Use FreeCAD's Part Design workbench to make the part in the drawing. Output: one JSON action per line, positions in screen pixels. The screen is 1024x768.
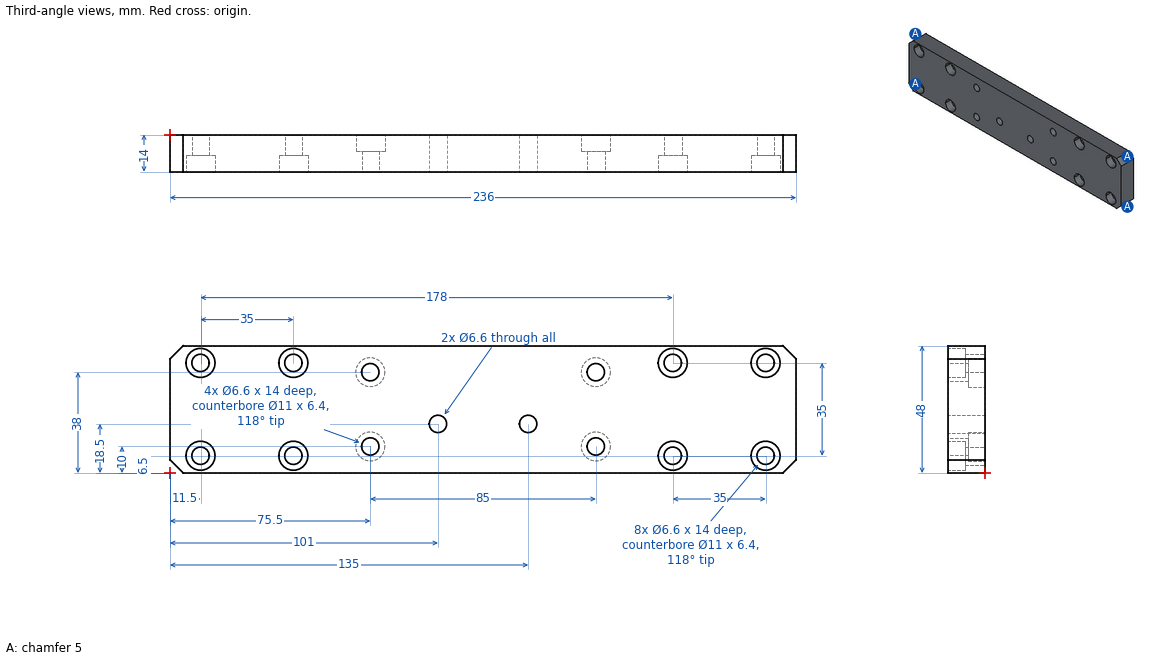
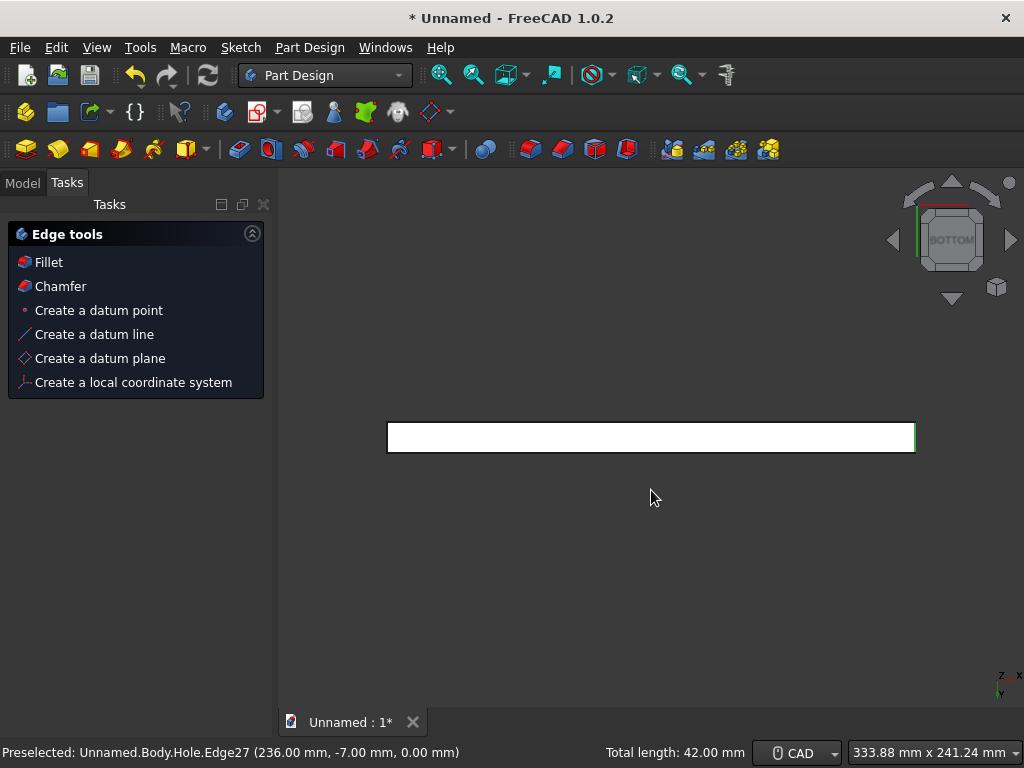
{"action": "left_click", "coordinate": [387, 436], "text": "ctrl"}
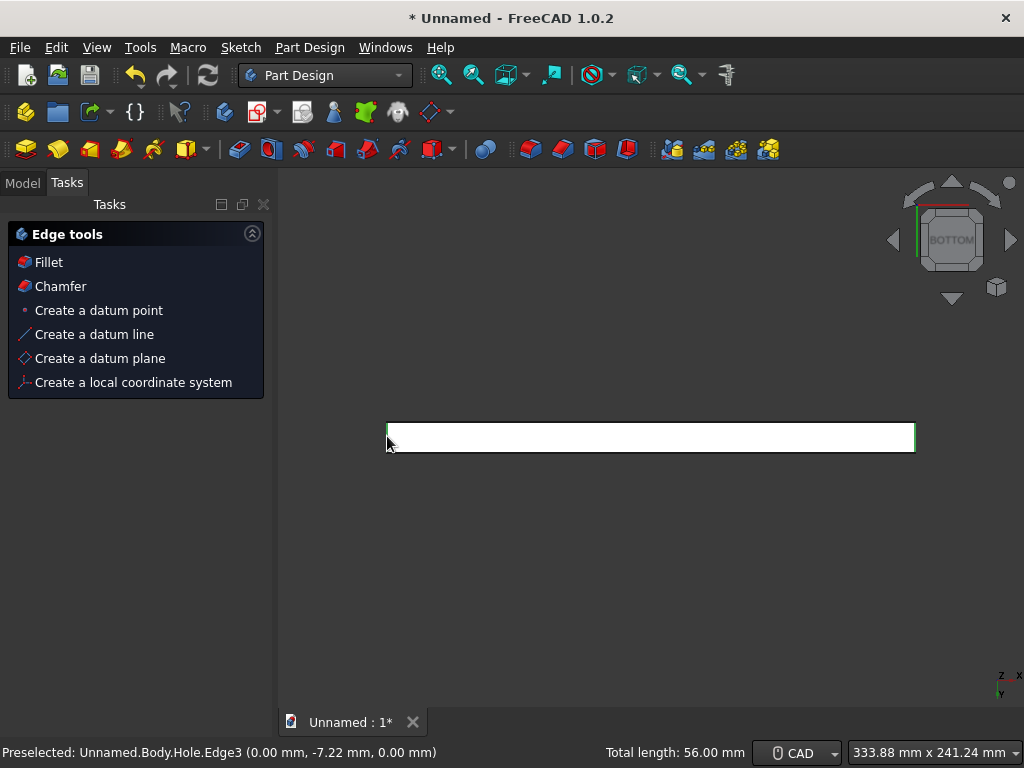
{"action": "left_click", "coordinate": [564, 150]}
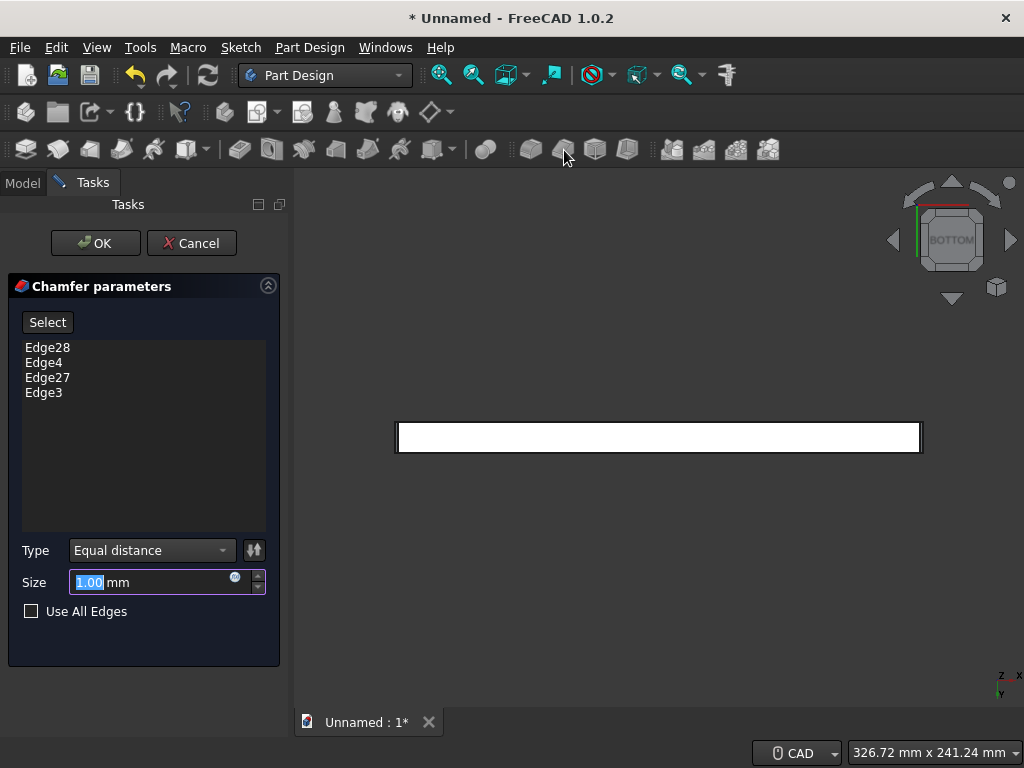
{"action": "type", "text": "5"}
{"action": "key", "text": "Tab"}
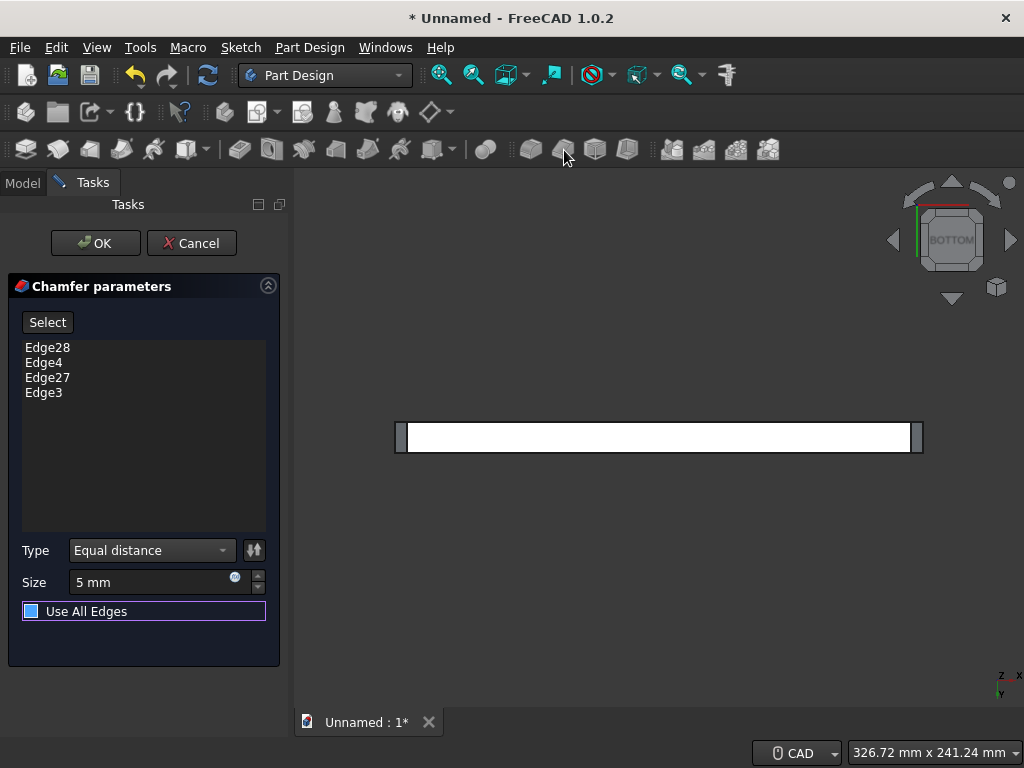
{"action": "left_click", "coordinate": [96, 243]}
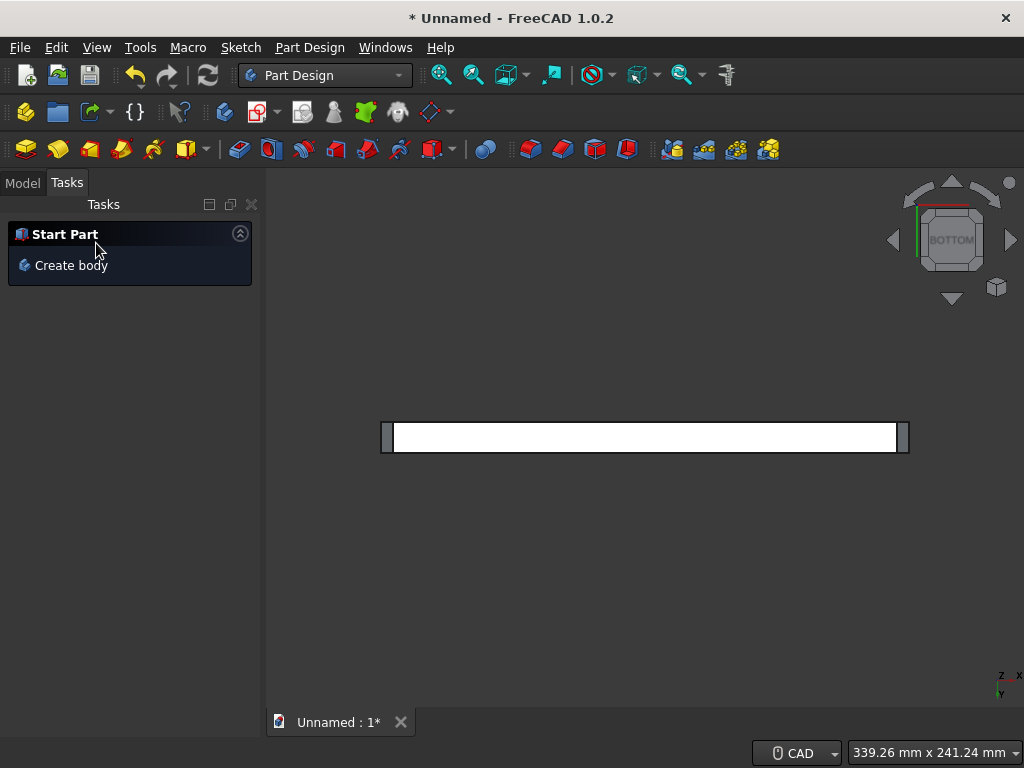
{"action": "key", "text": "4"}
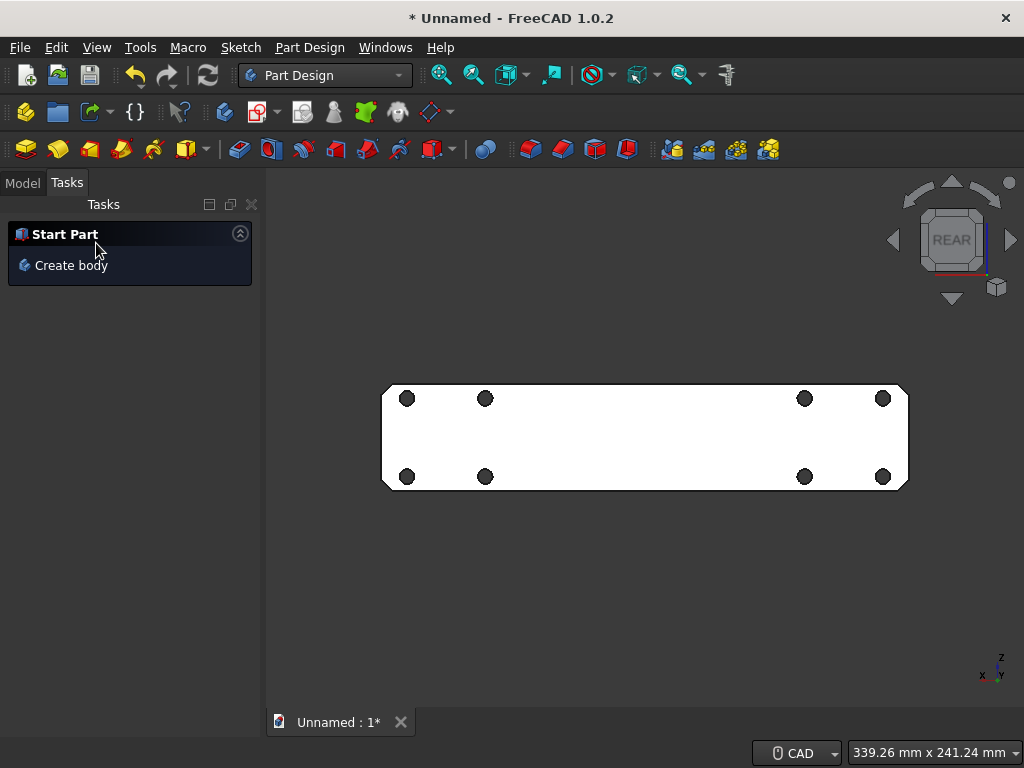
{"action": "left_click", "coordinate": [570, 437]}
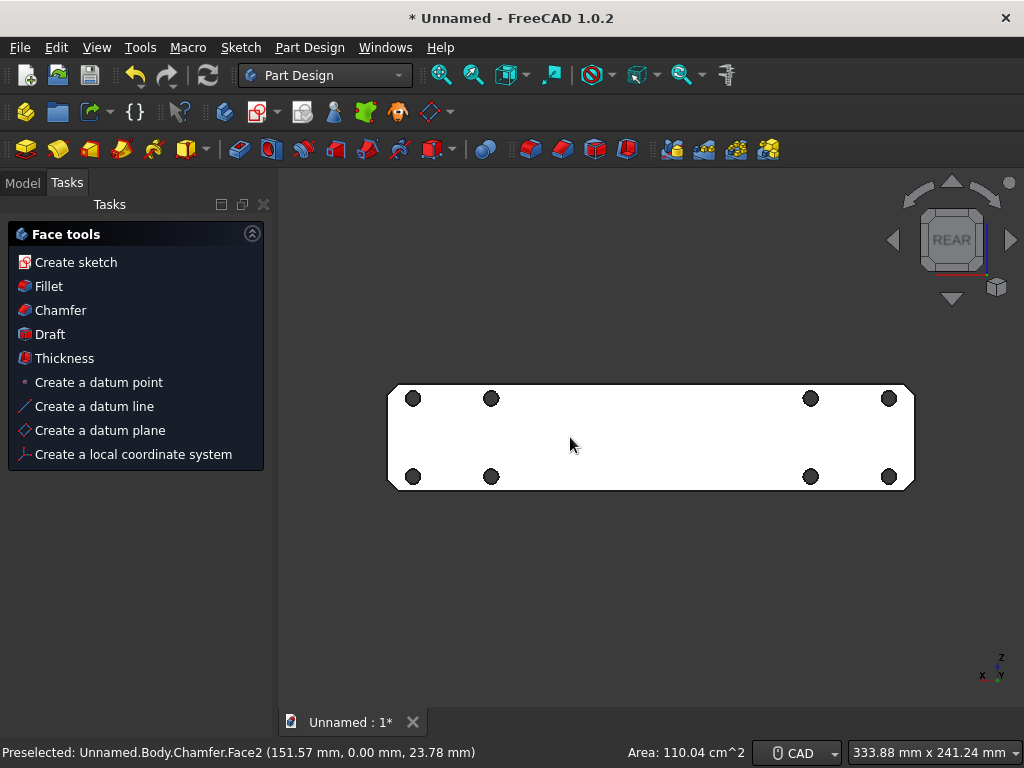
{"action": "left_click", "coordinate": [258, 112]}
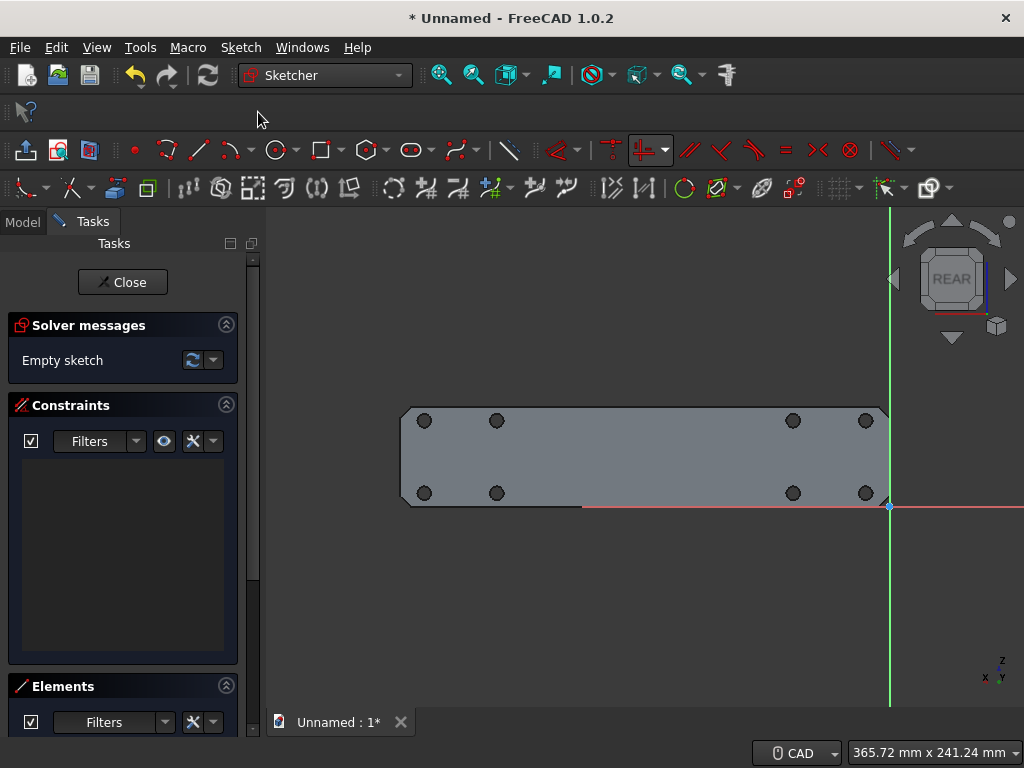
{"action": "scroll", "coordinate": [294, 426], "scroll_direction": "down", "scroll_amount": 1}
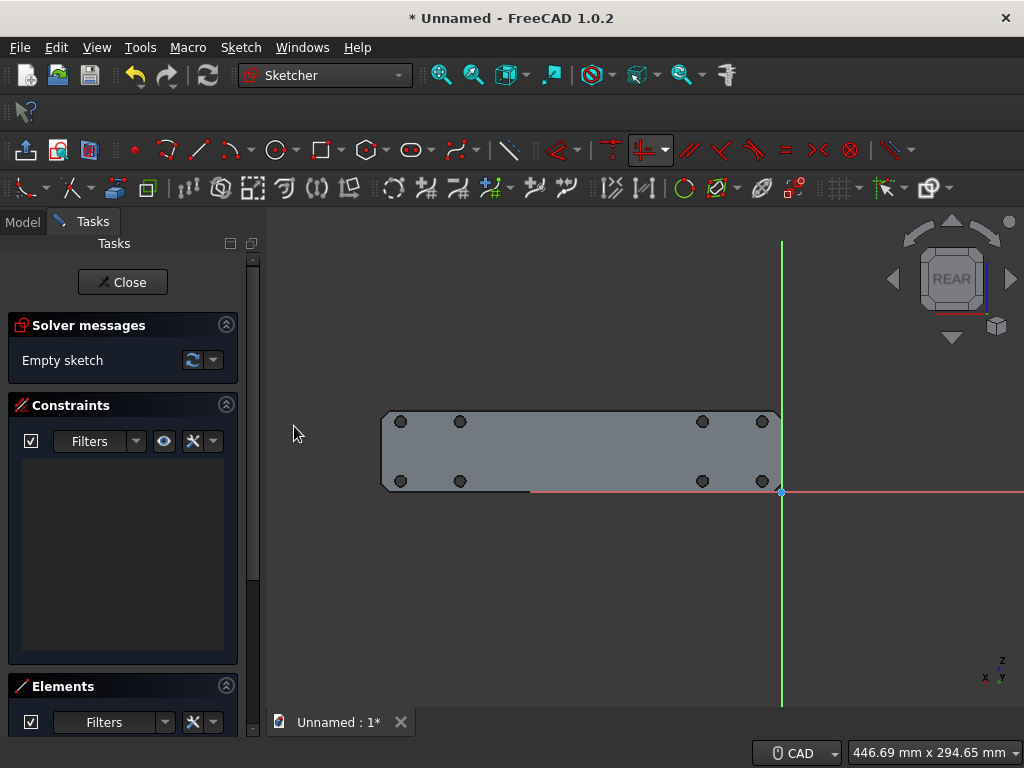
{"action": "scroll", "coordinate": [777, 457], "scroll_direction": "up", "scroll_amount": 2}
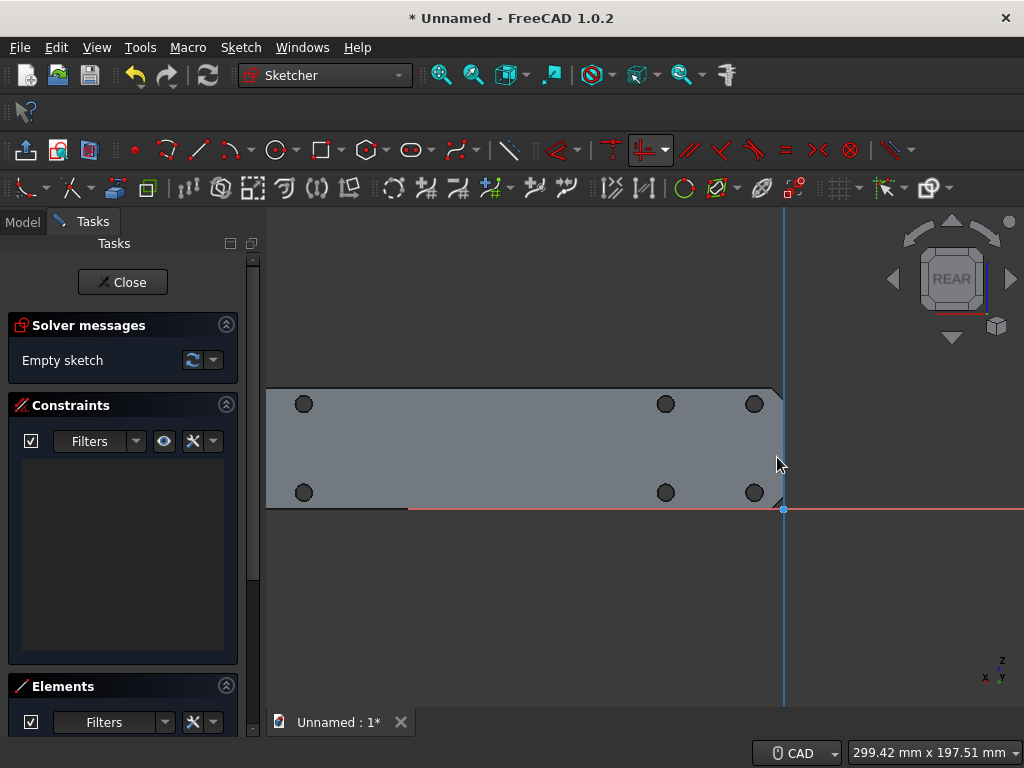
{"action": "left_click", "coordinate": [276, 150]}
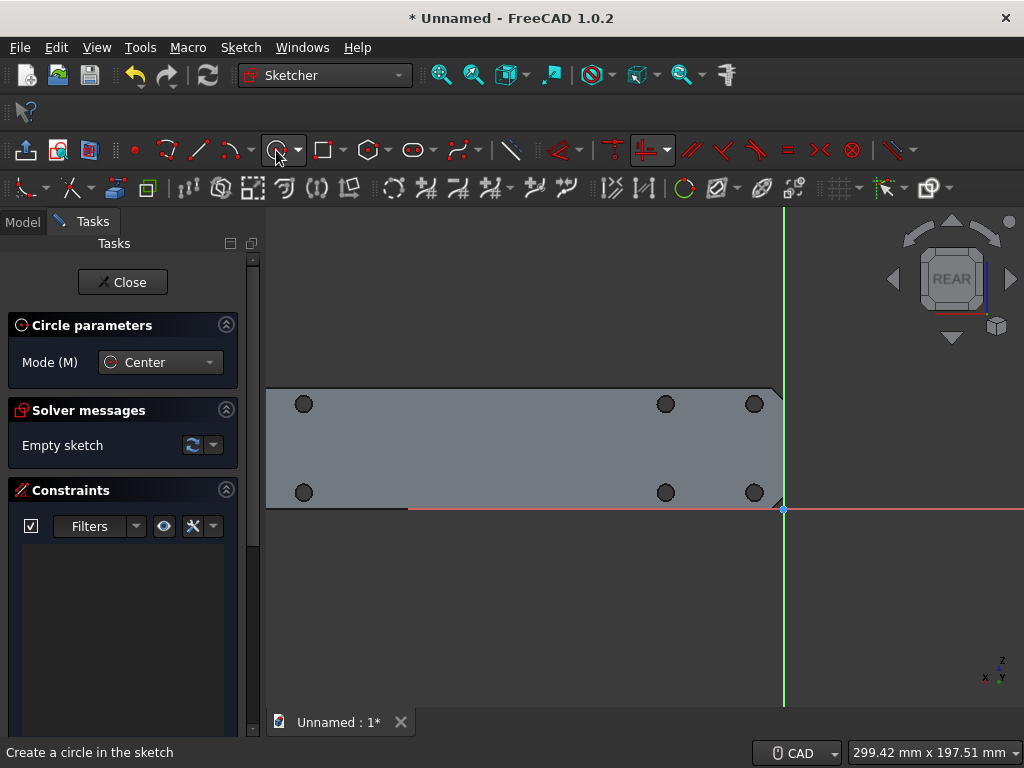
{"action": "scroll", "coordinate": [592, 484], "scroll_direction": "up", "scroll_amount": 5}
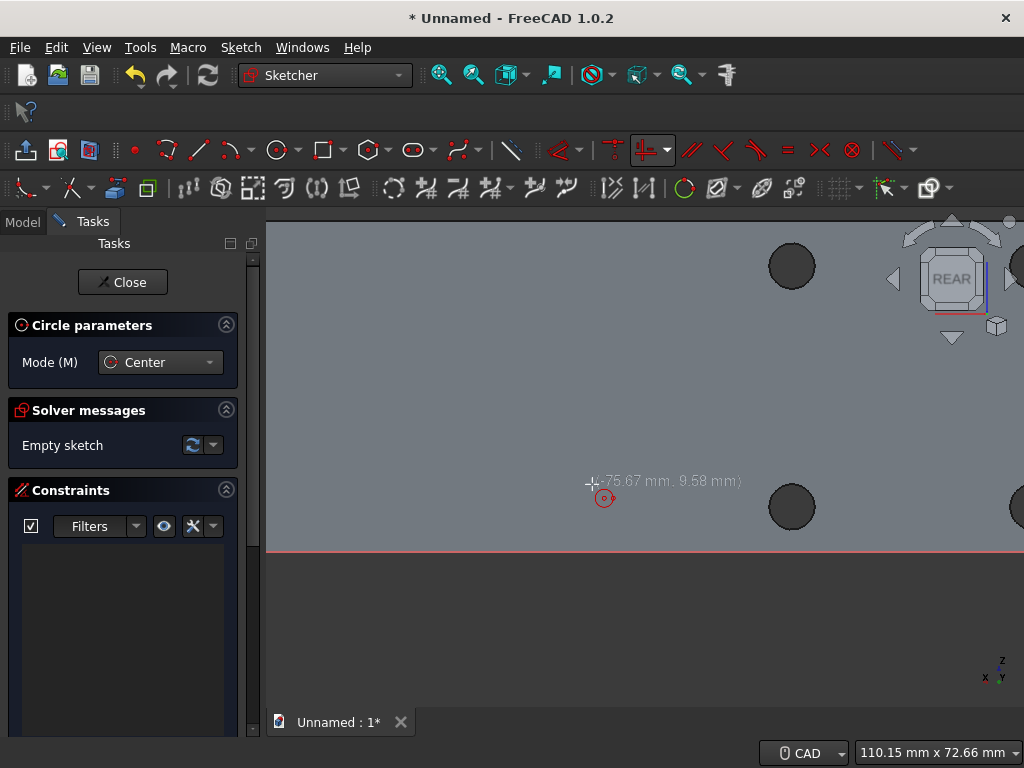
{"action": "left_click", "coordinate": [592, 483]}
{"action": "left_click", "coordinate": [608, 467]}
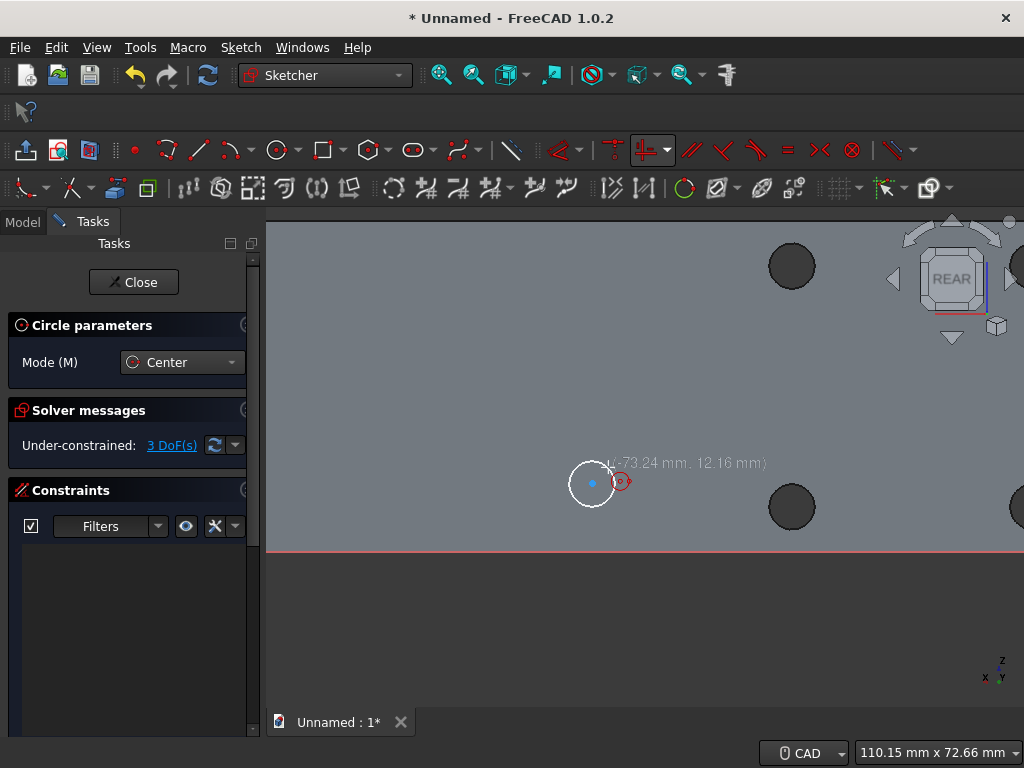
{"action": "scroll", "coordinate": [593, 485], "scroll_direction": "down", "scroll_amount": 5}